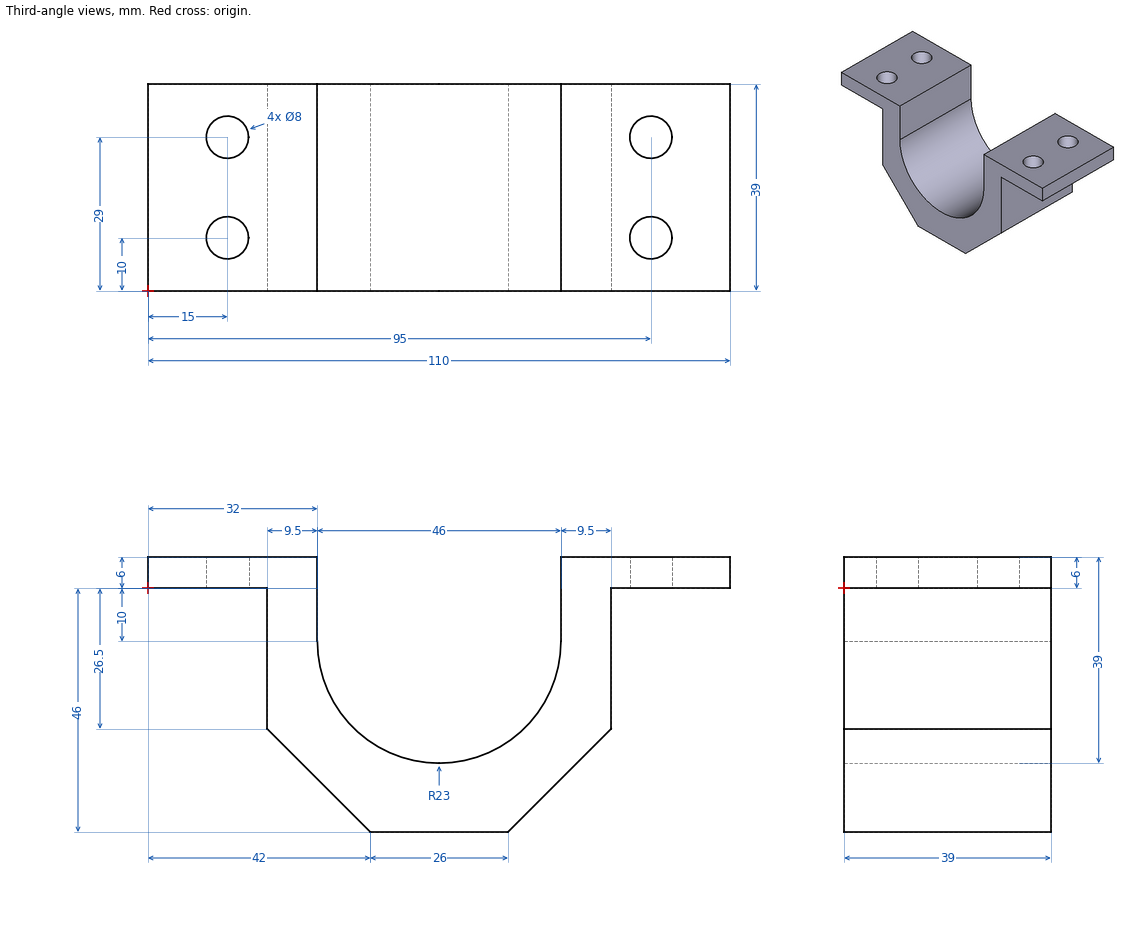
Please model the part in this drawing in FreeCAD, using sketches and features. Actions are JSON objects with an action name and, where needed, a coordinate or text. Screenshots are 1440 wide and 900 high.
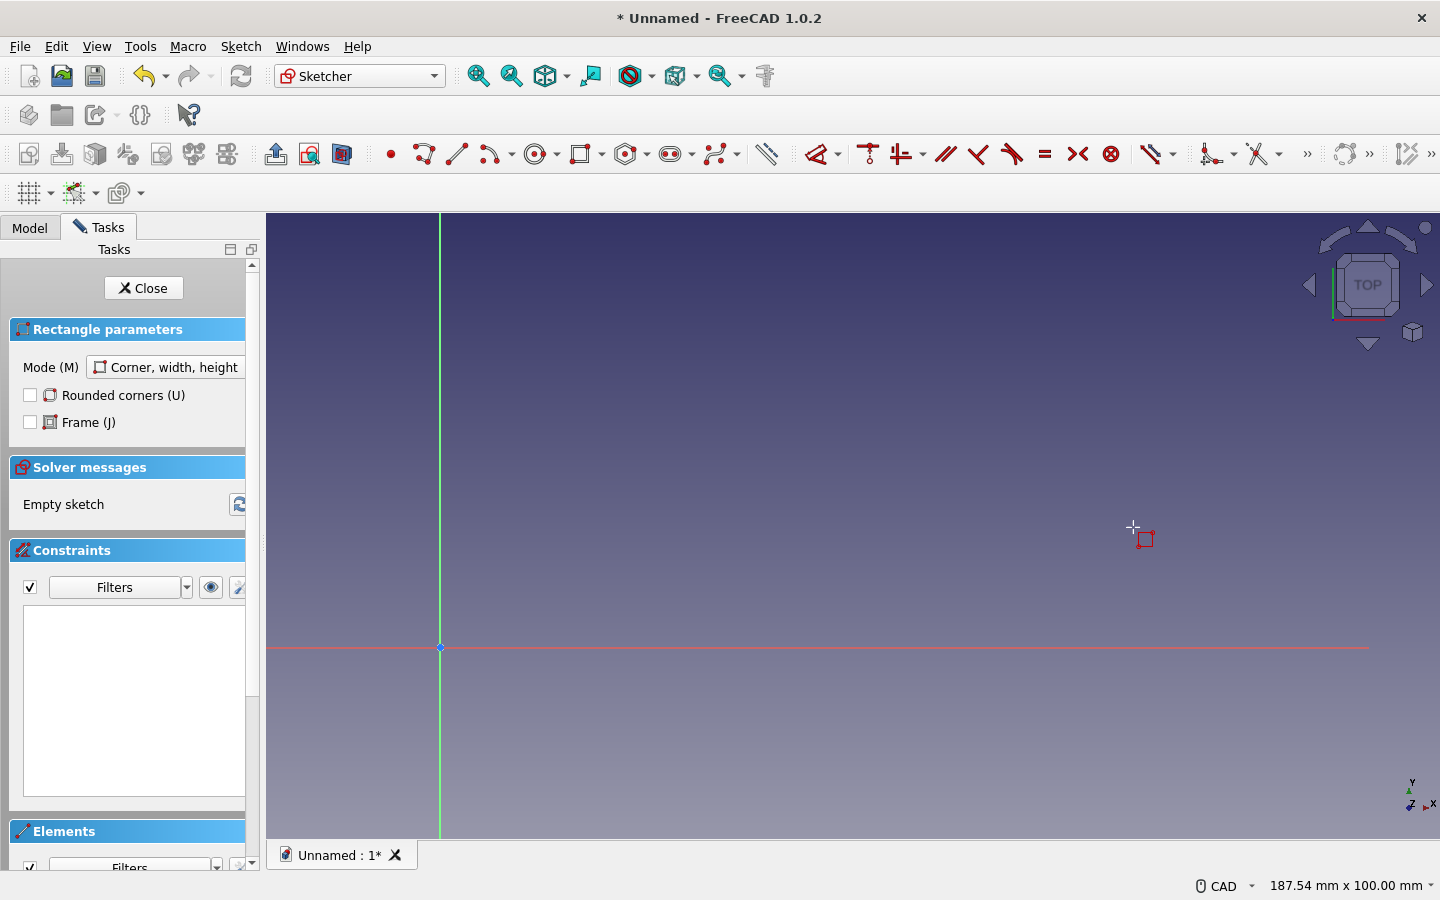
{"action": "left_click", "coordinate": [440, 648]}
{"action": "left_click", "coordinate": [1129, 404]}
{"action": "key", "text": "Escape"}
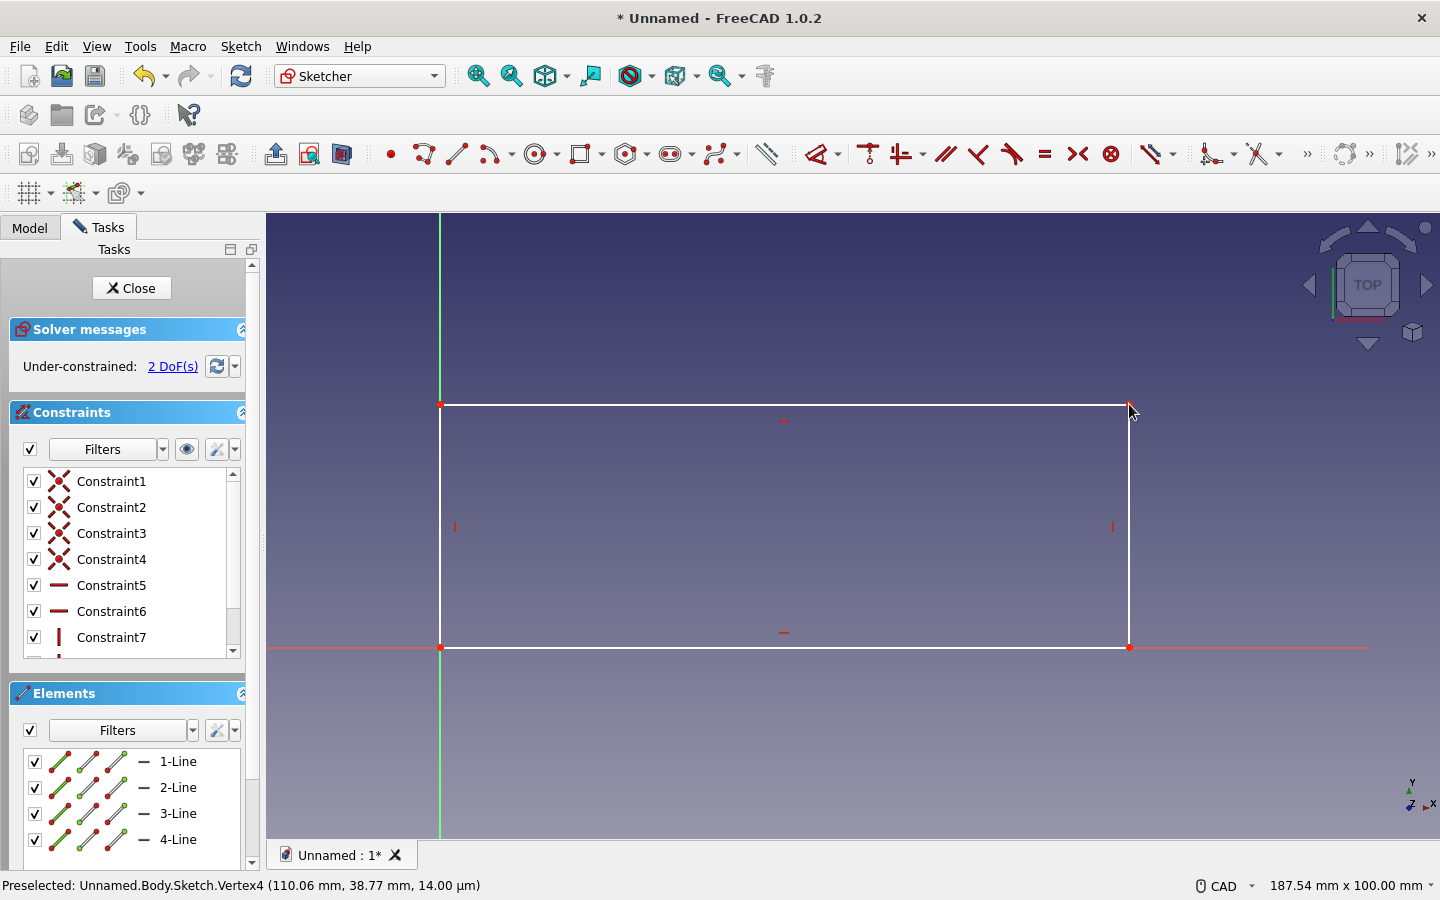
{"action": "key", "text": "d"}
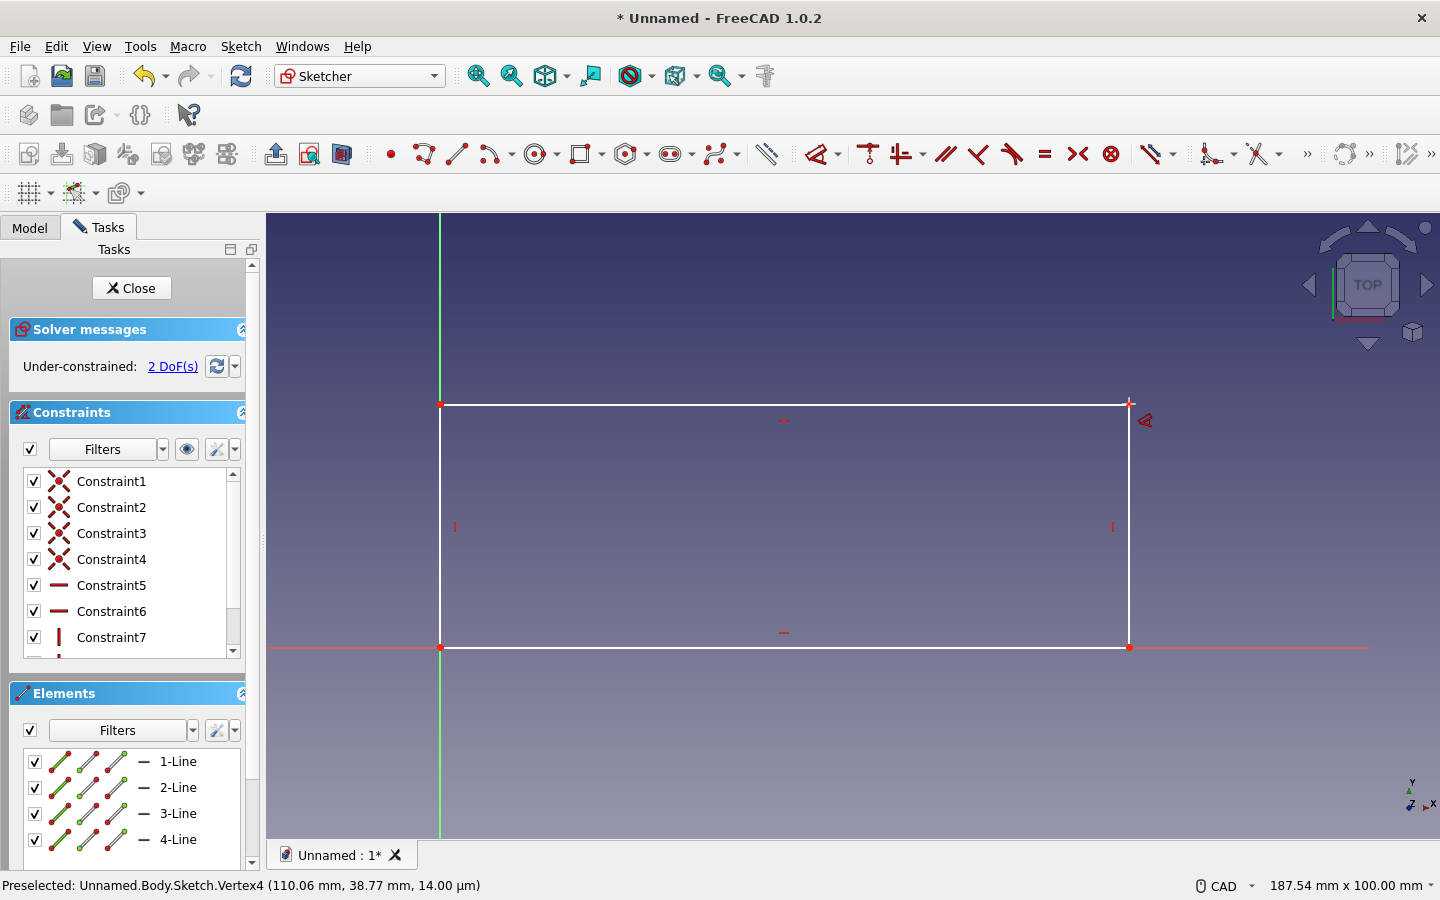
{"action": "left_click", "coordinate": [1129, 575]}
{"action": "left_click", "coordinate": [1163, 526]}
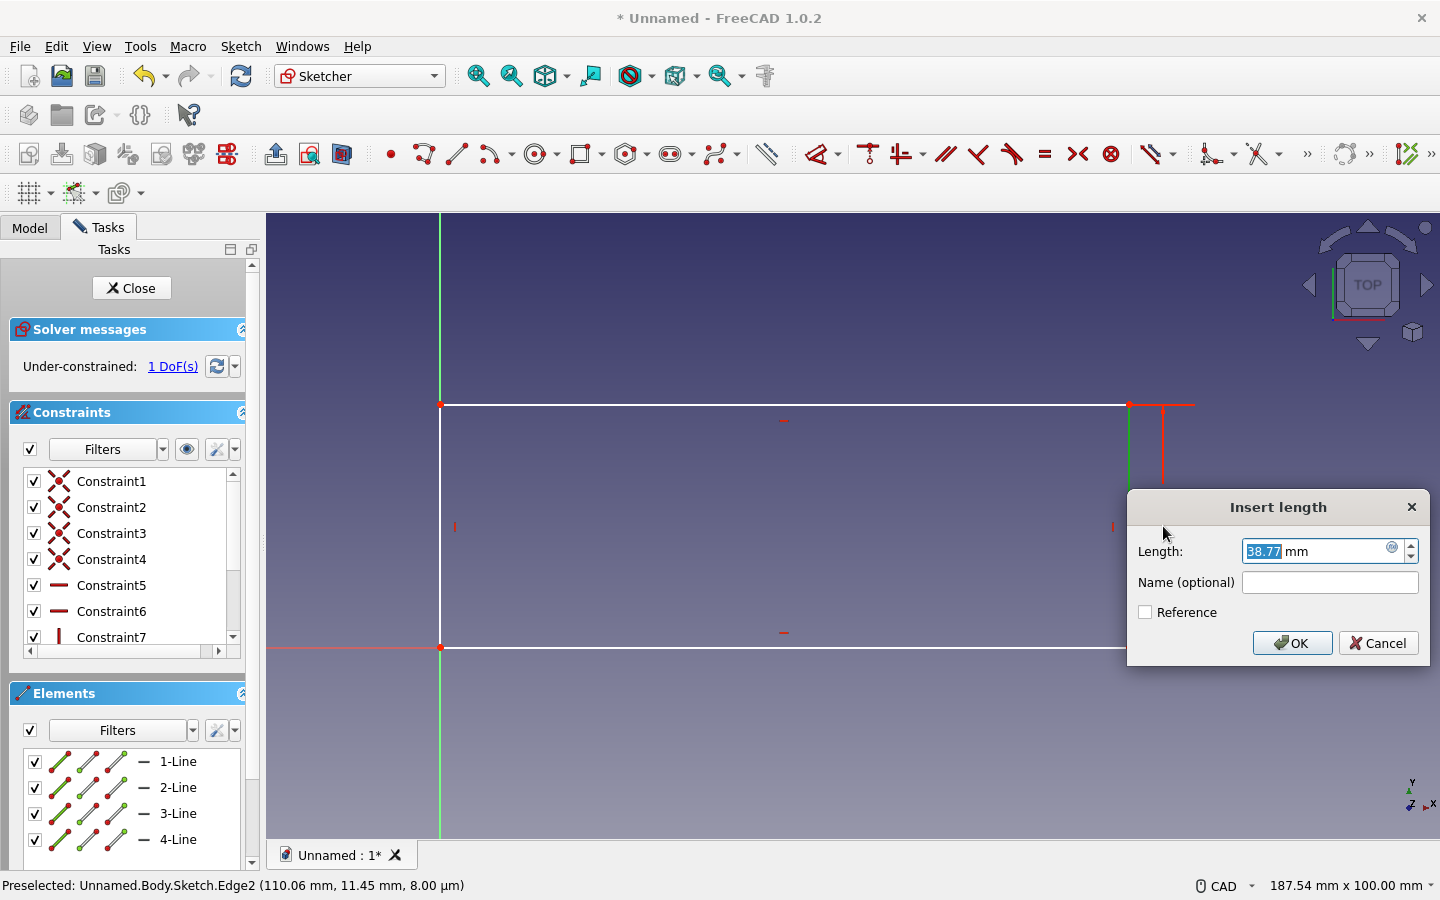
{"action": "type", "text": "39"}
{"action": "key", "text": "Return"}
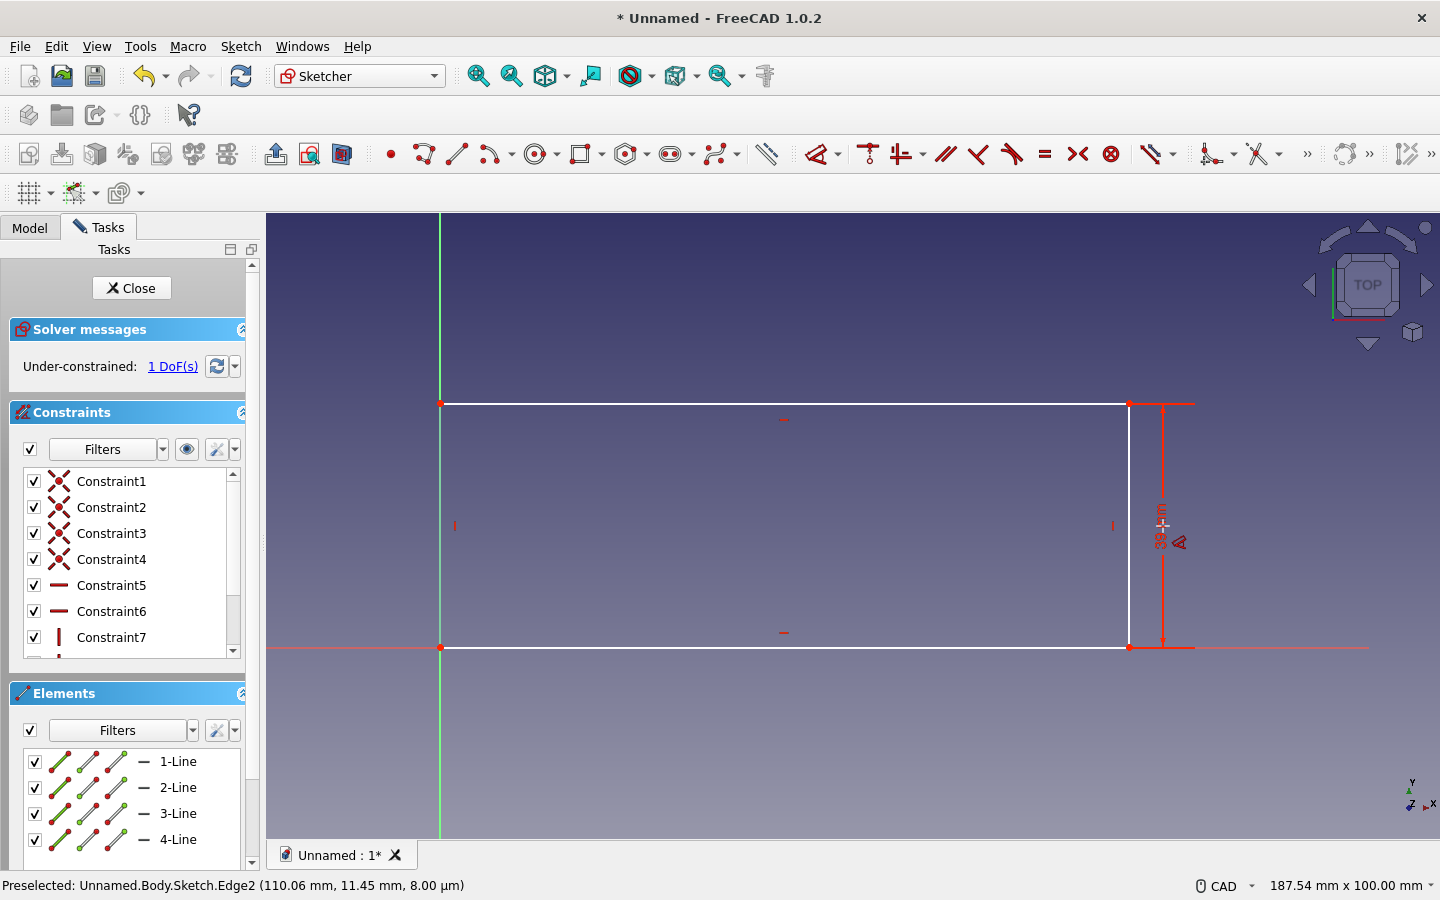
{"action": "left_click", "coordinate": [647, 648]}
{"action": "left_click", "coordinate": [785, 682]}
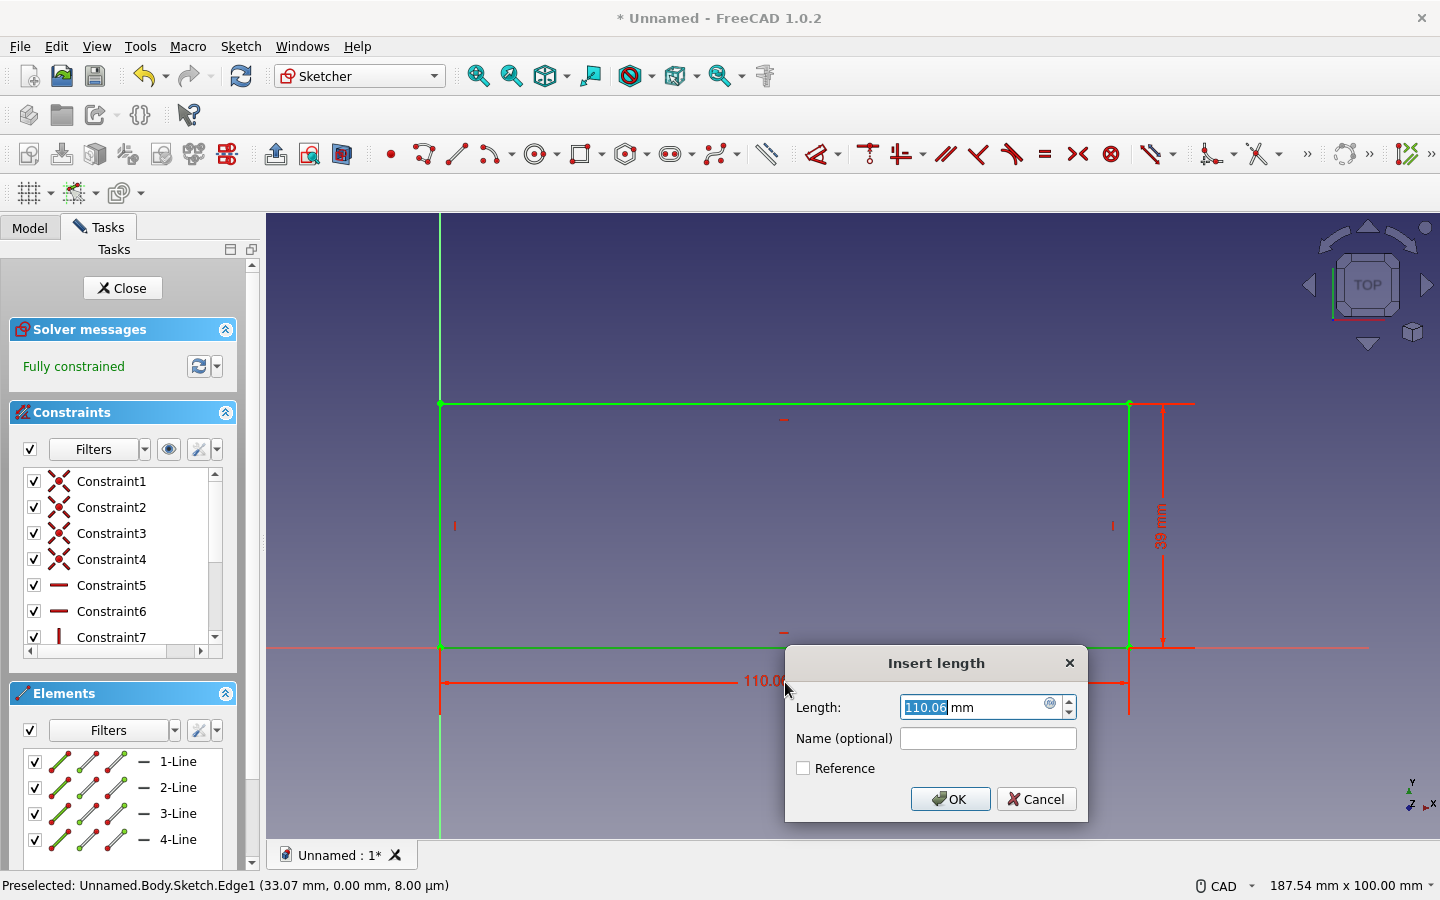
{"action": "type", "text": "110"}
{"action": "key", "text": "Return"}
{"action": "key", "text": "Escape"}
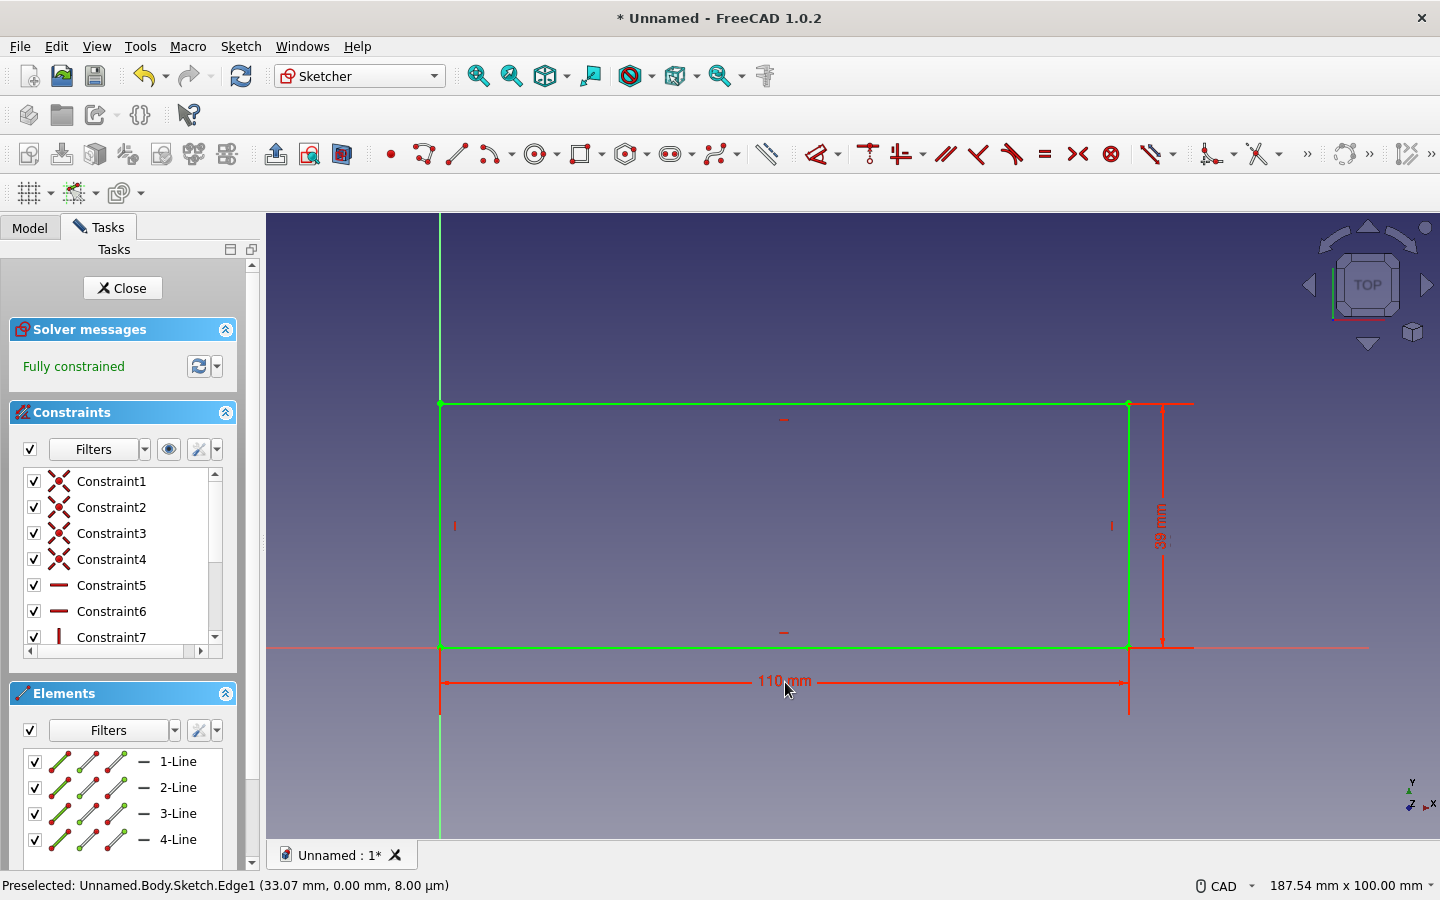
{"action": "left_click", "coordinate": [123, 288]}